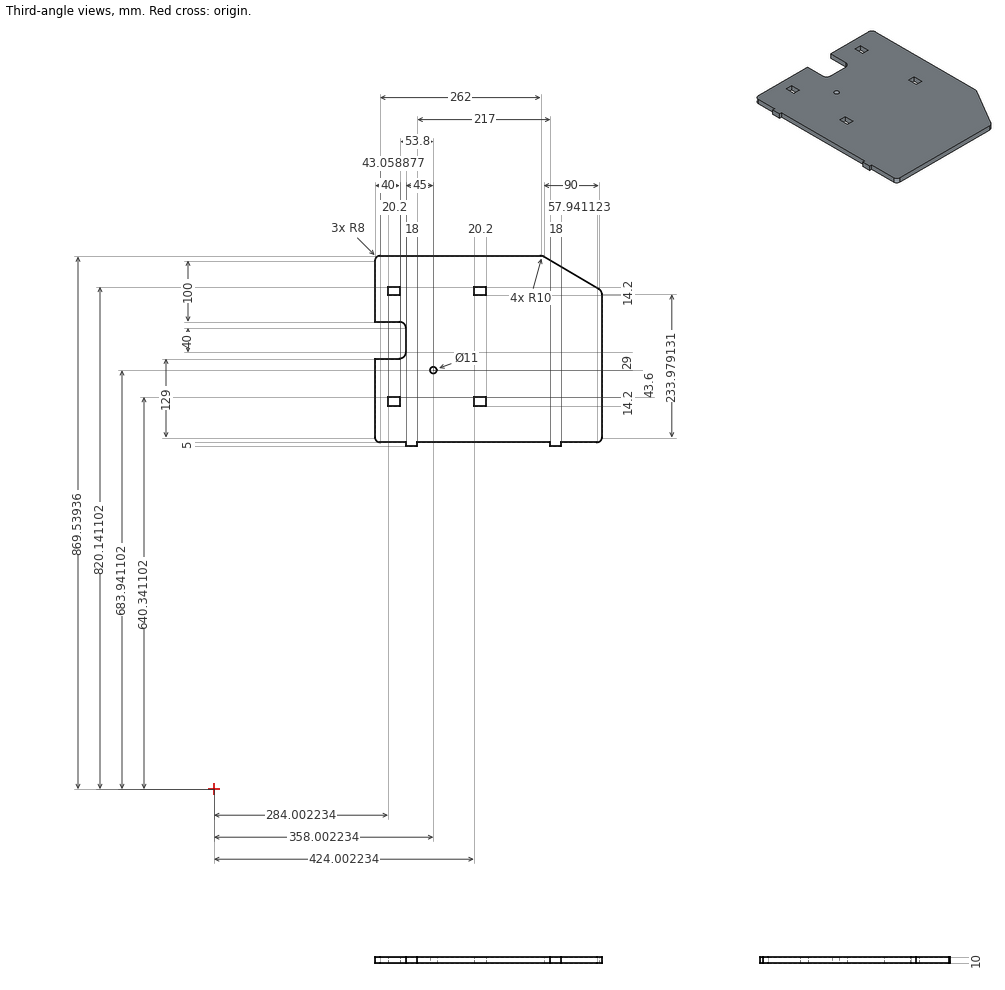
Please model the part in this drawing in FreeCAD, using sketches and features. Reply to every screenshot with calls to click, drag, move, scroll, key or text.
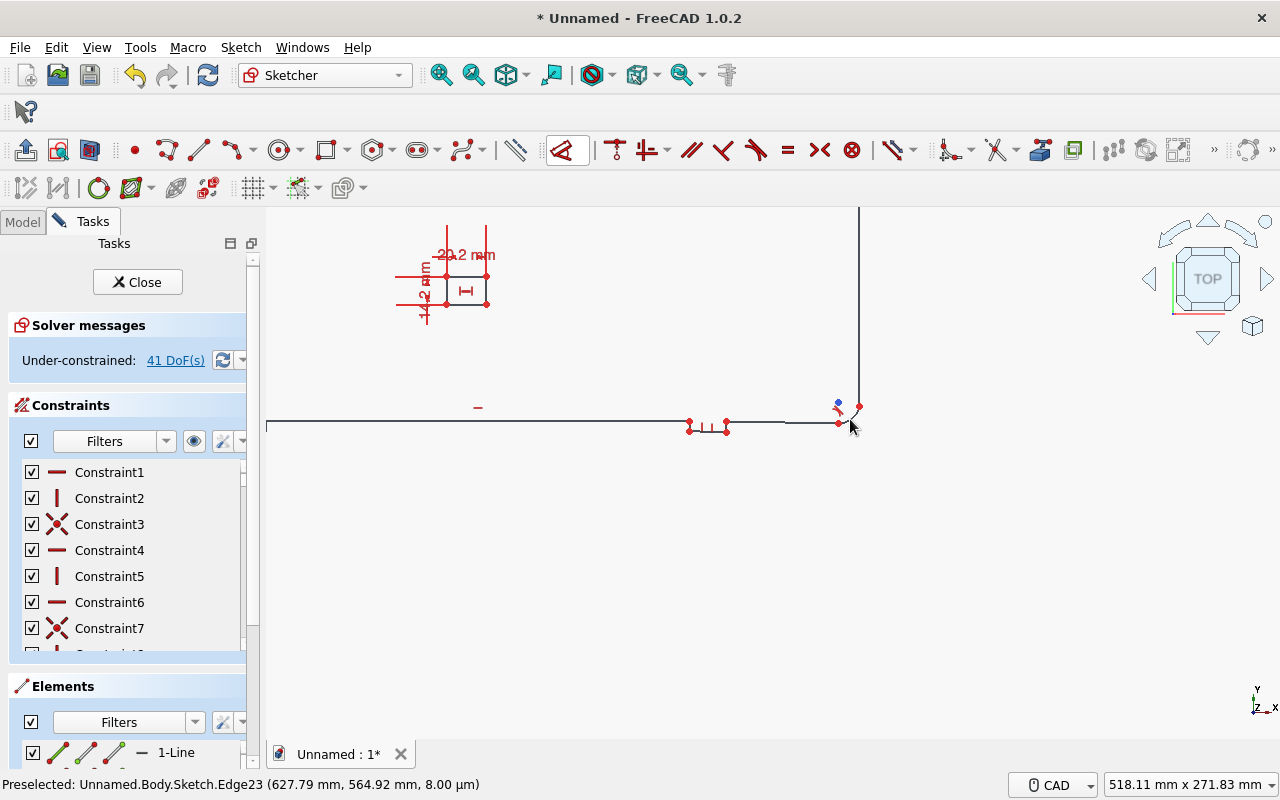
scroll(823, 422, down, 8)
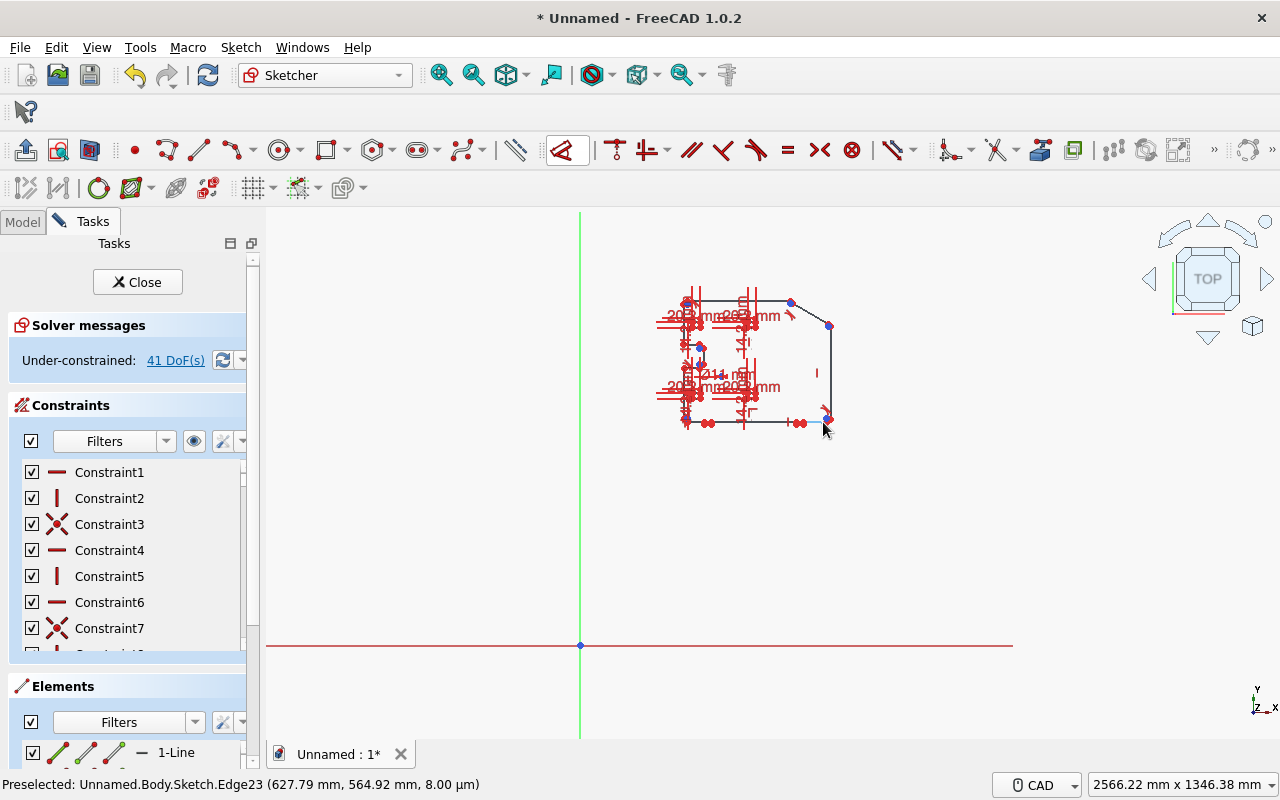
click(831, 391)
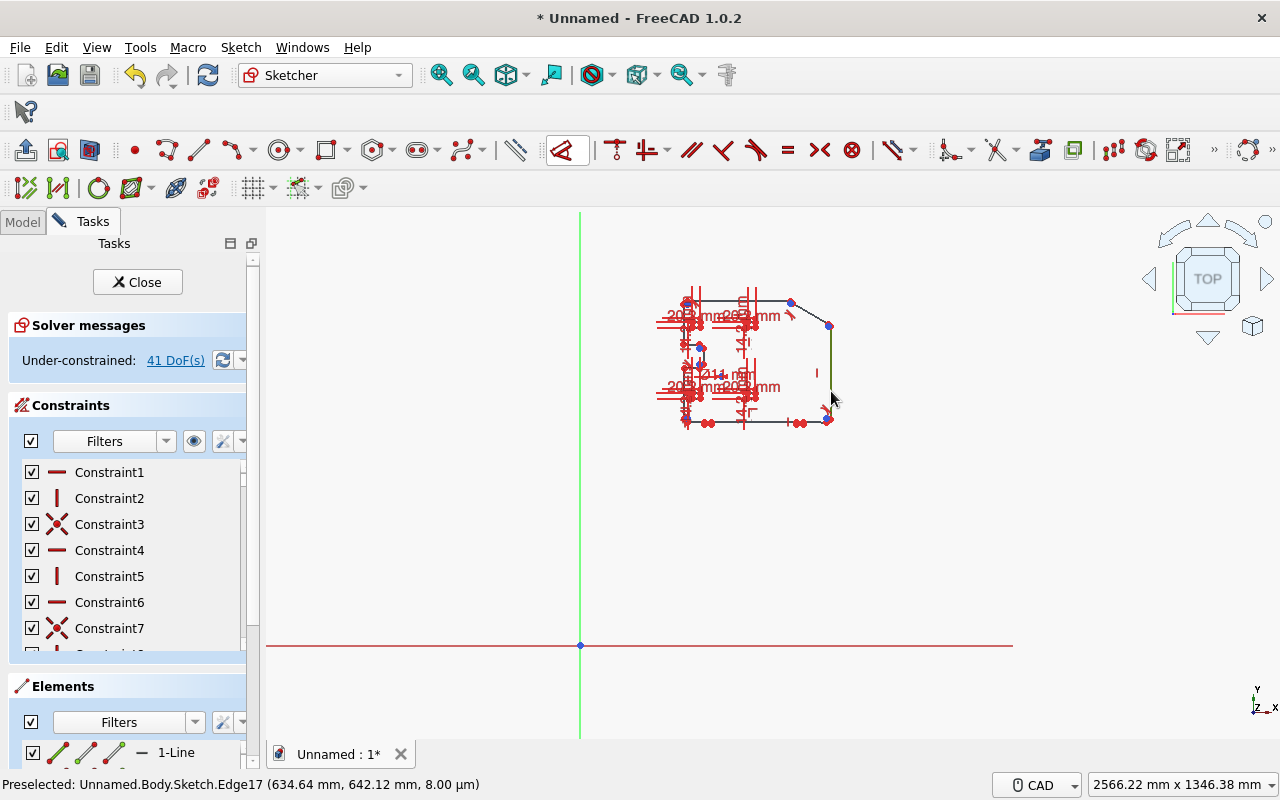
scroll(829, 422, up, 8)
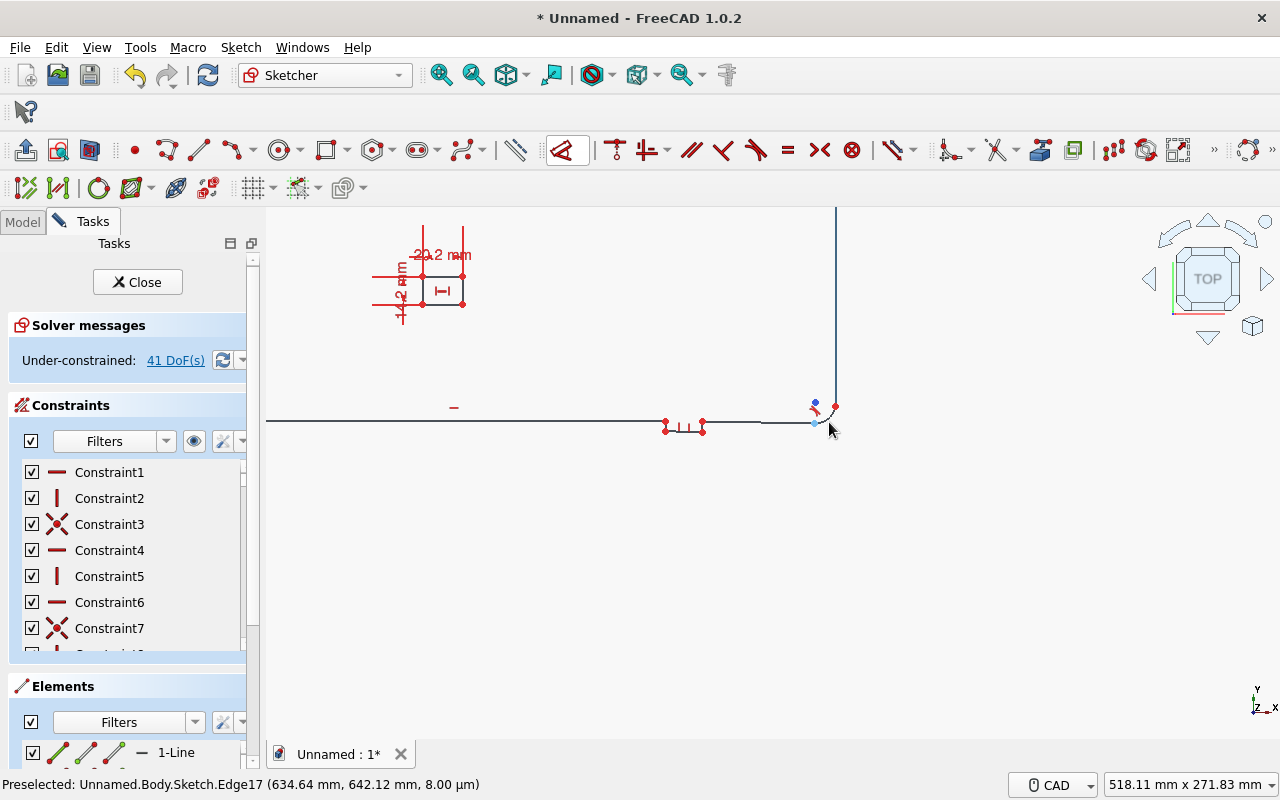
click(828, 419)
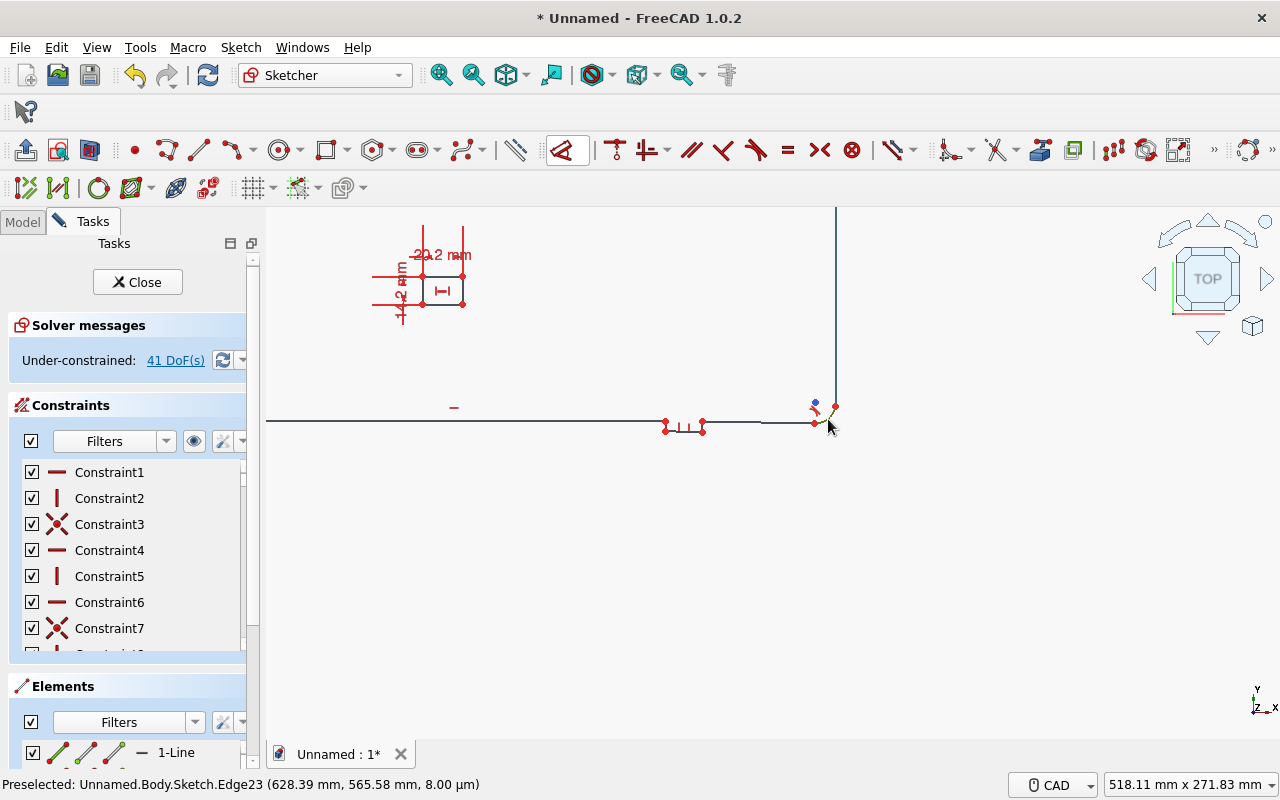
click(756, 150)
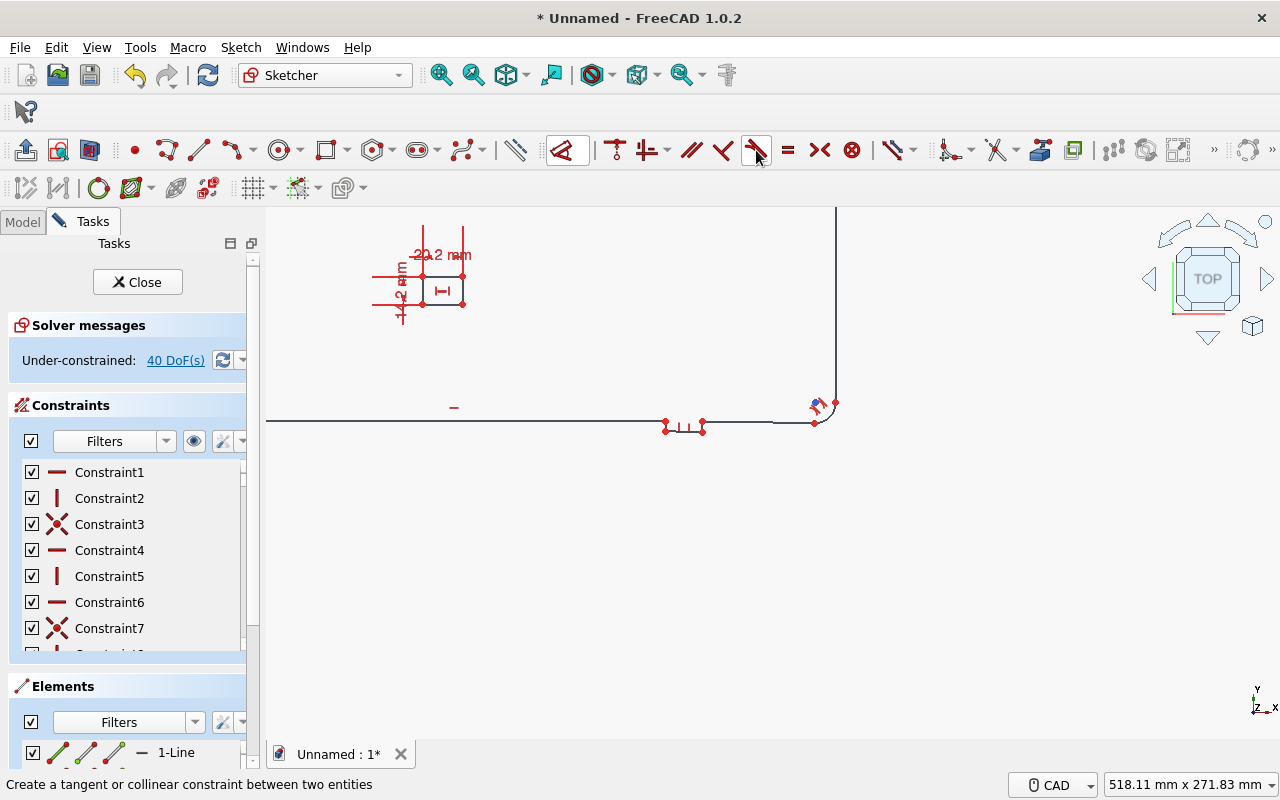
scroll(829, 422, down, 8)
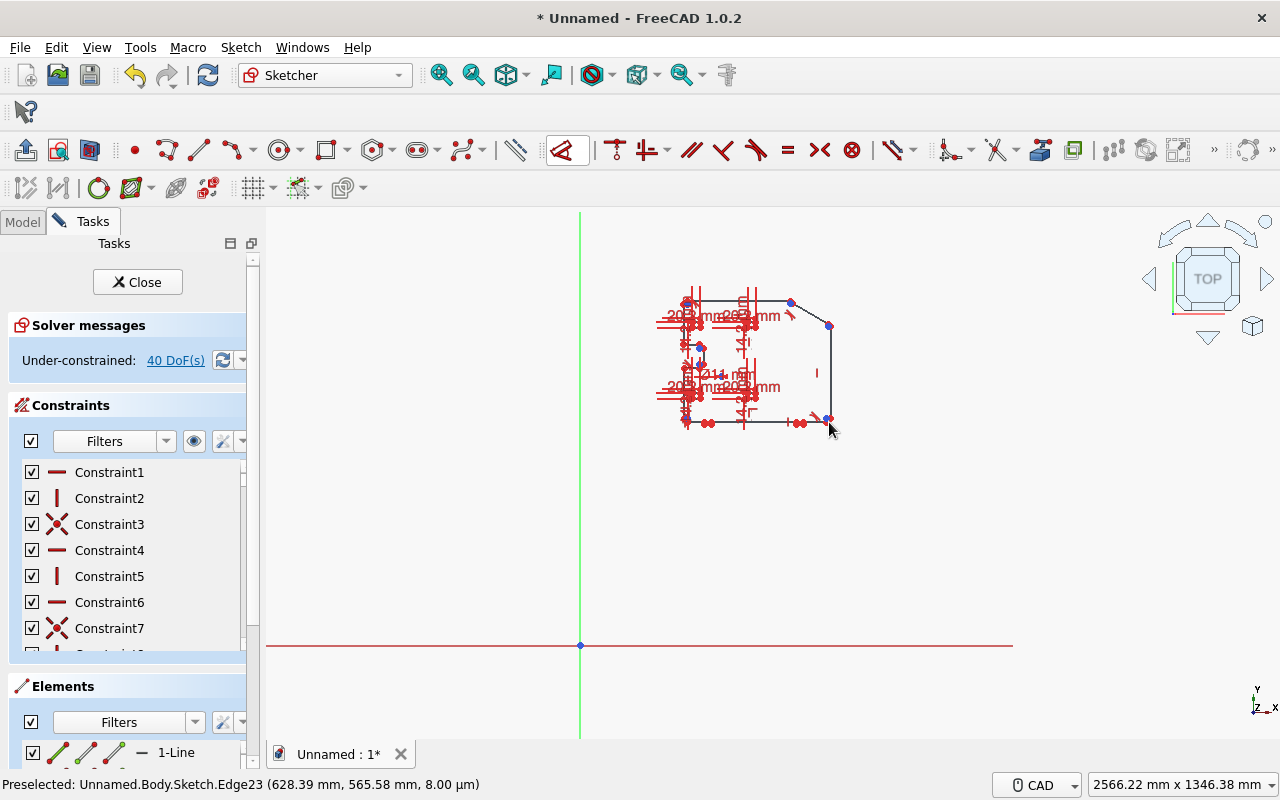
click(831, 391)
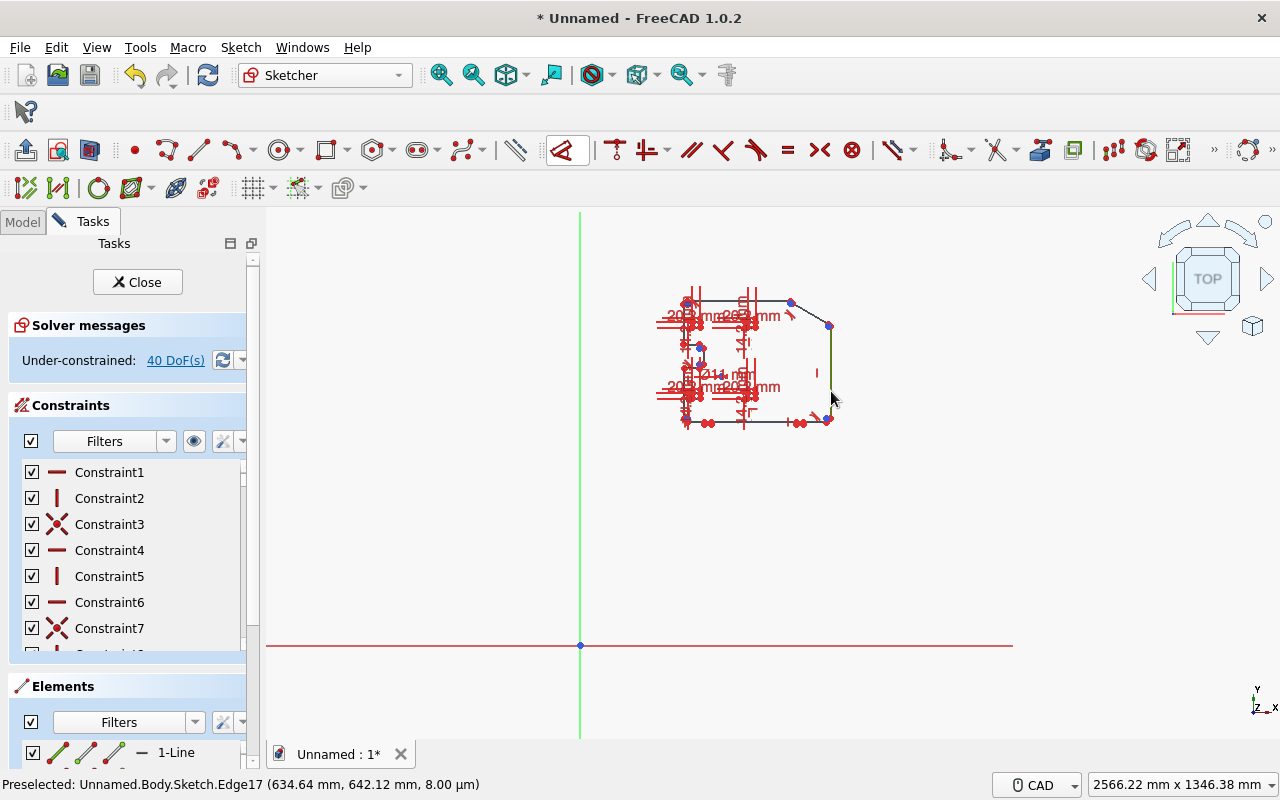
scroll(830, 325, up, 10)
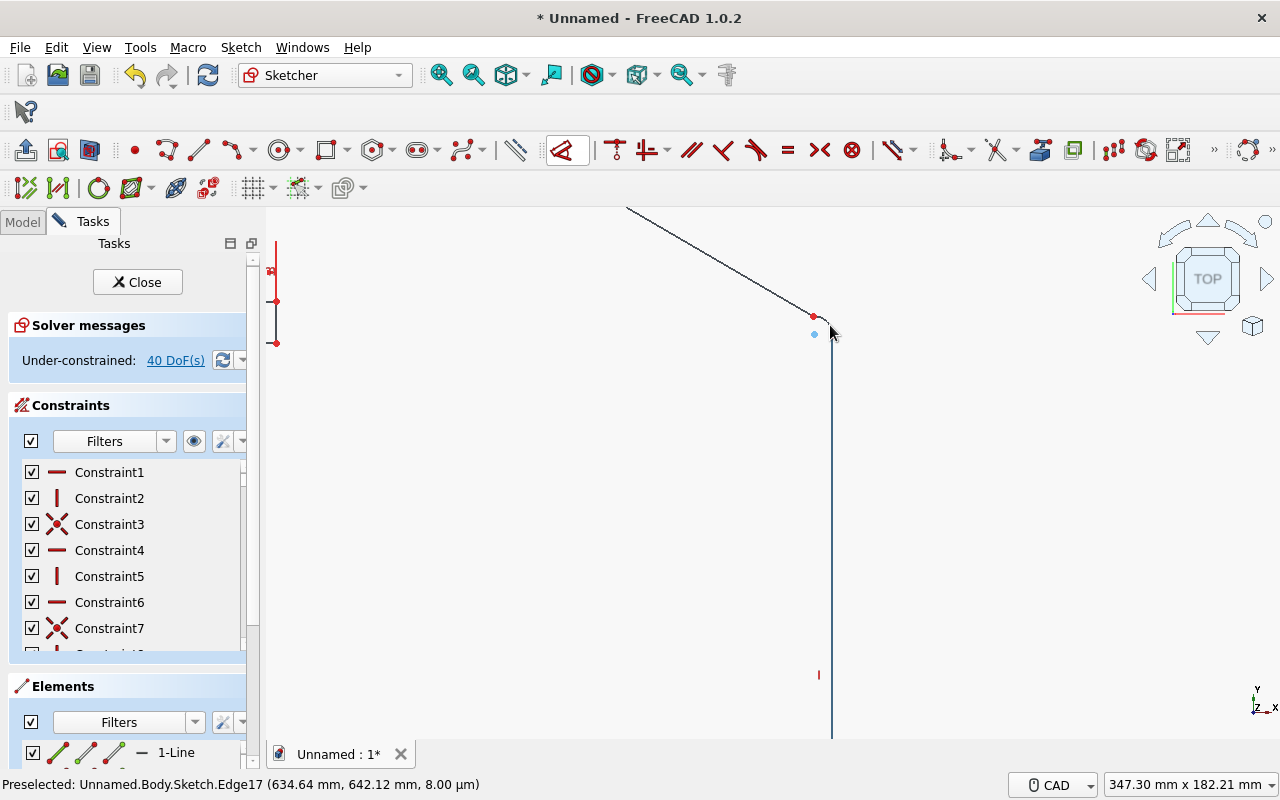
click(827, 322)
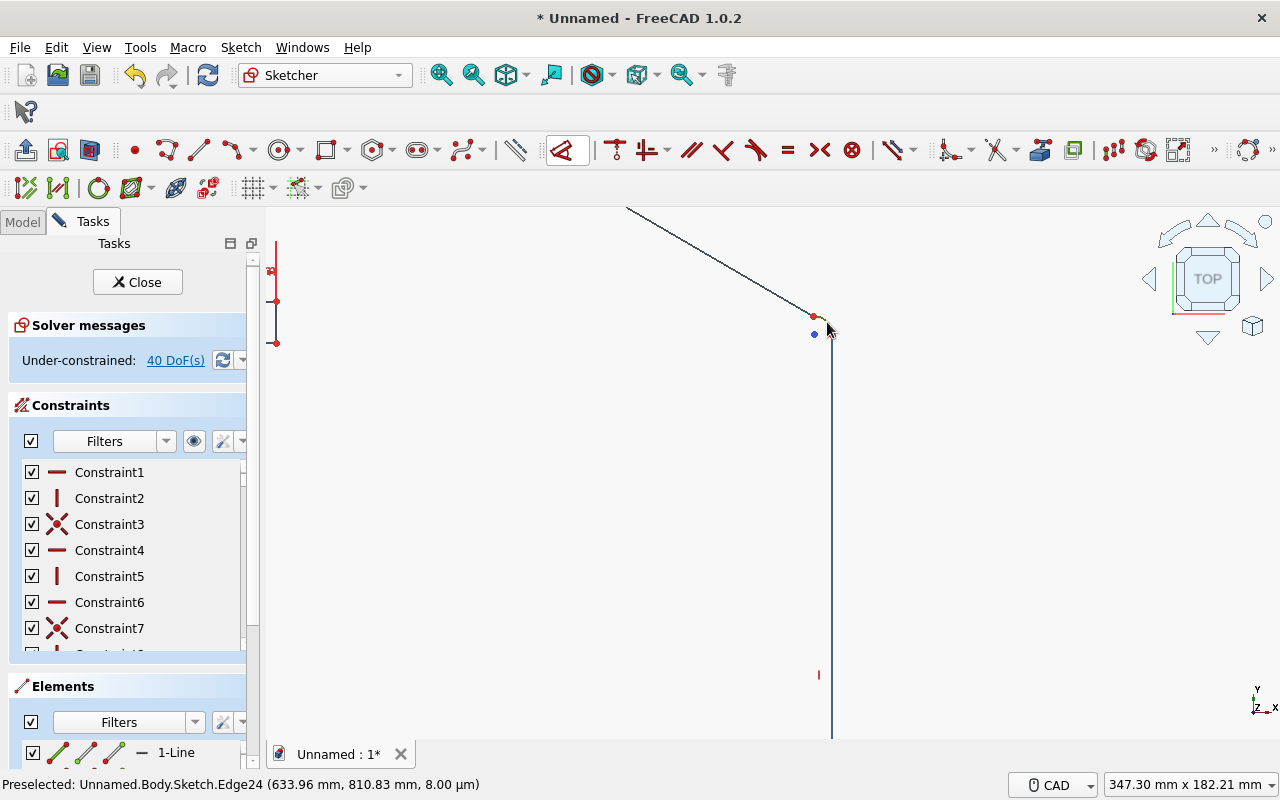
click(756, 150)